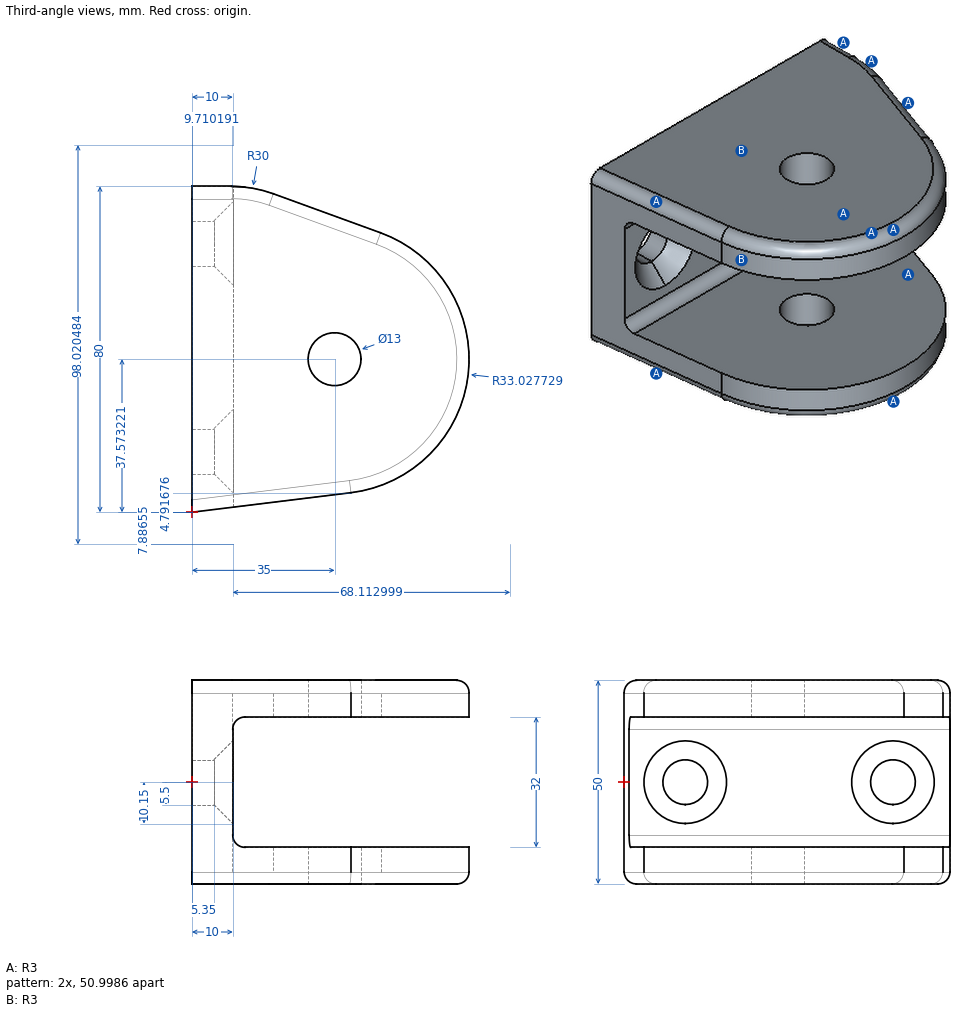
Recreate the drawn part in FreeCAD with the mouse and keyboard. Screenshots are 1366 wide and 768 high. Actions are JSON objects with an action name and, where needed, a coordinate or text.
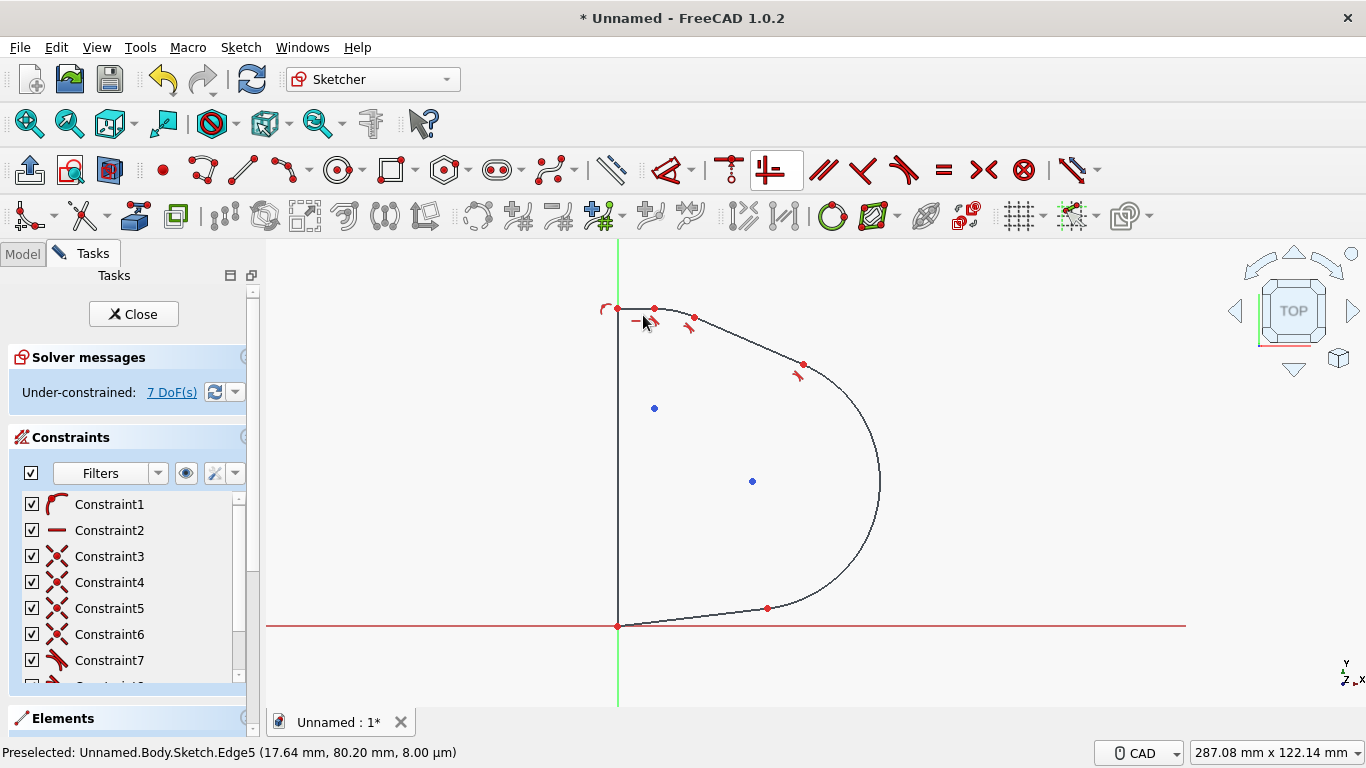
{"action": "left_click", "coordinate": [723, 614]}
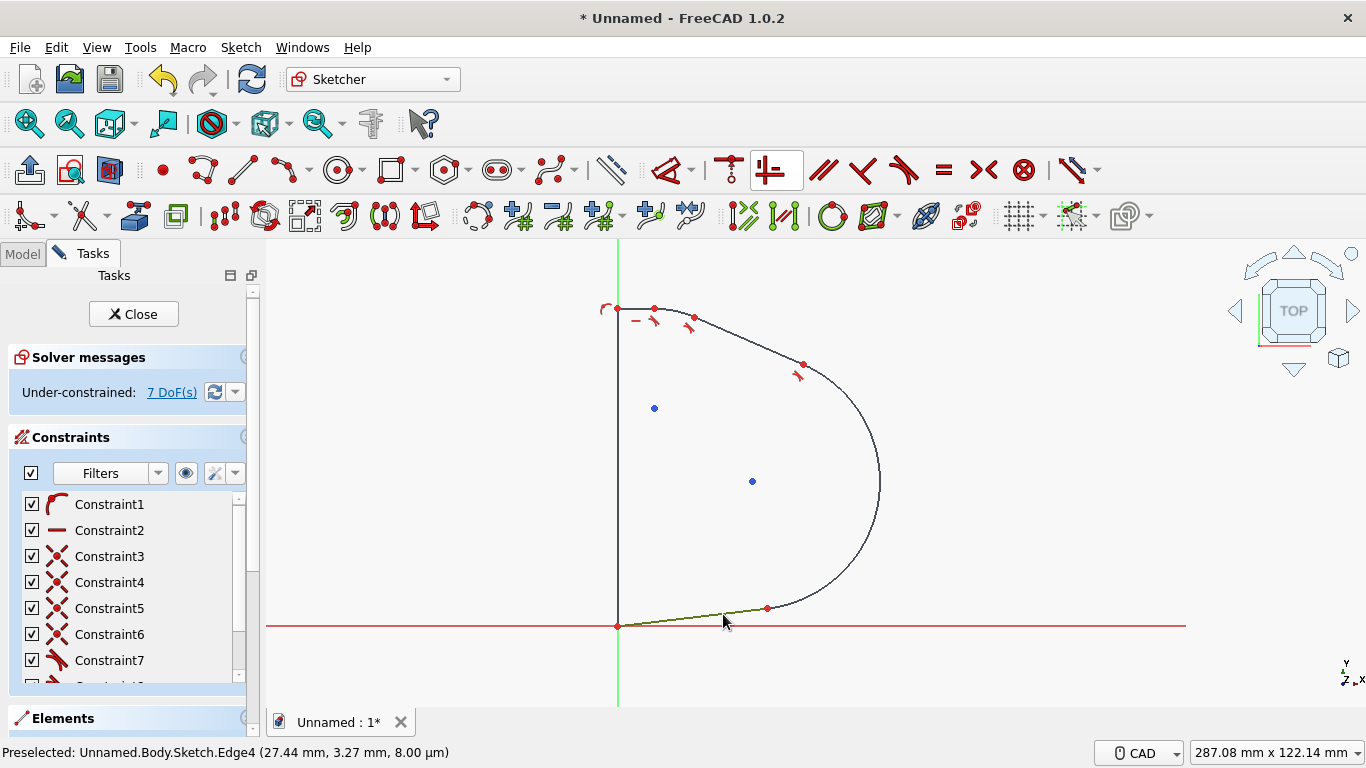
{"action": "left_click", "coordinate": [853, 561]}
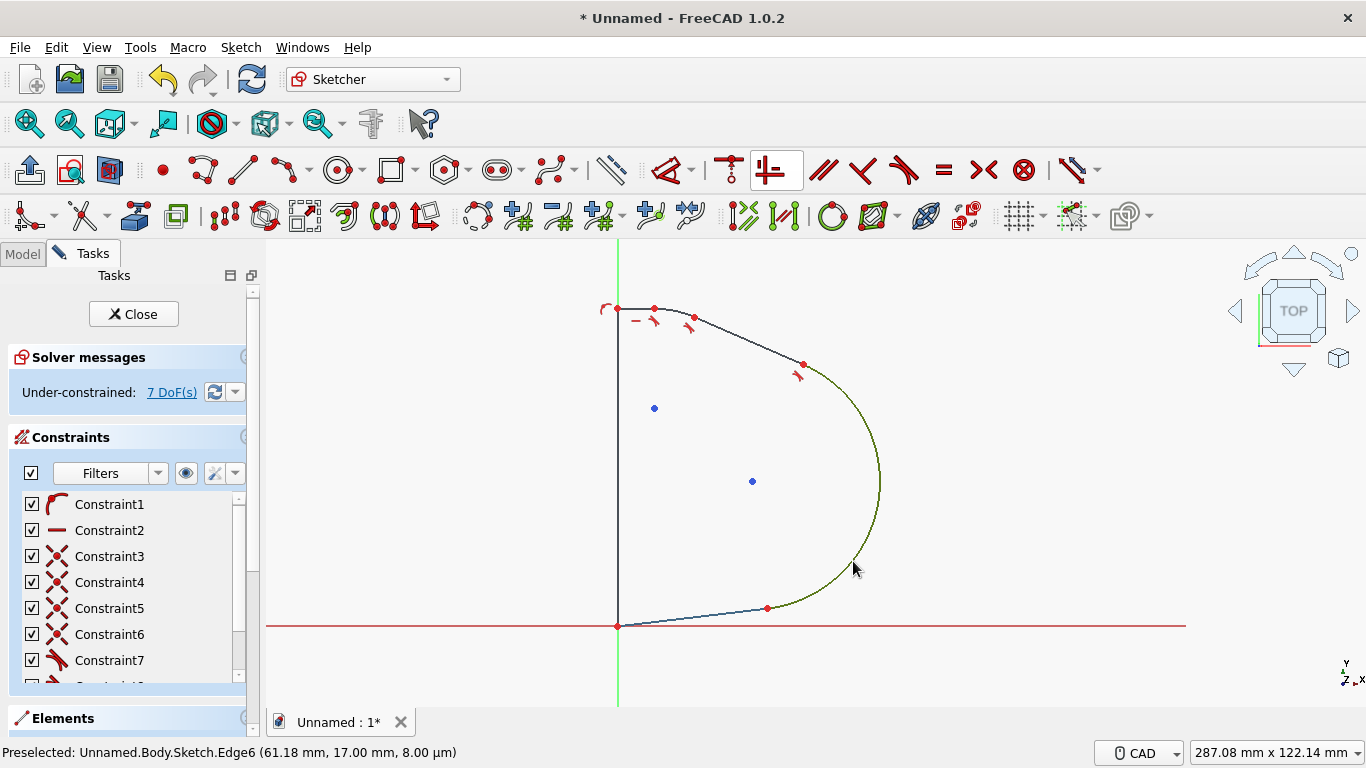
{"action": "left_click", "coordinate": [904, 170]}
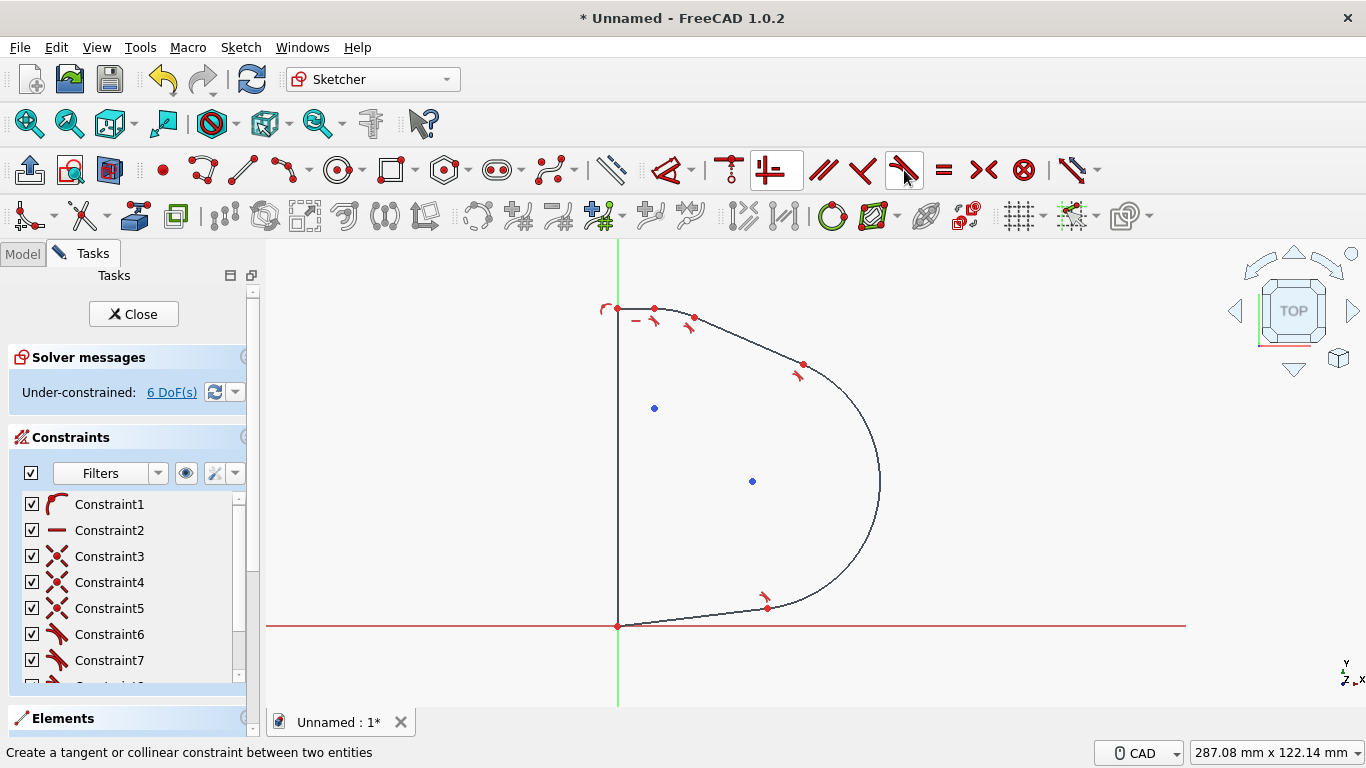
{"action": "left_click", "coordinate": [666, 170]}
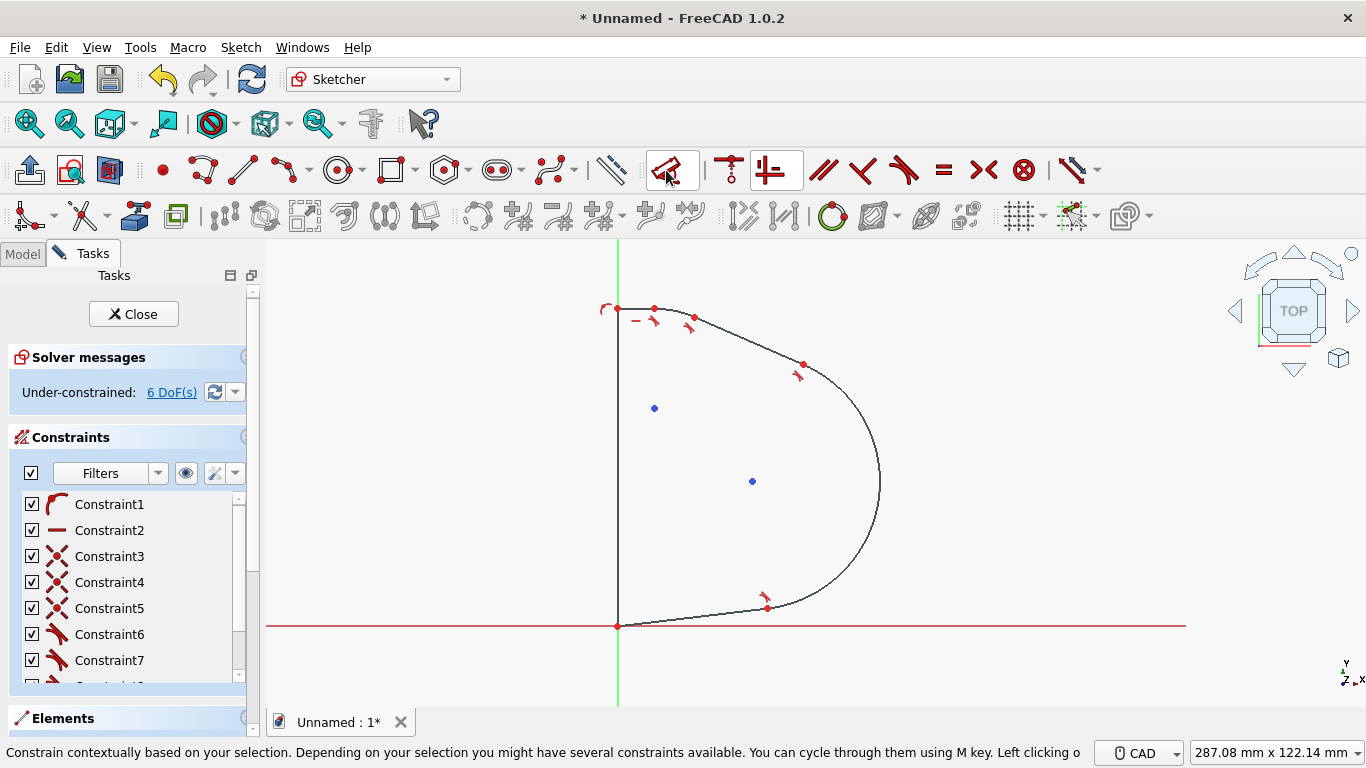
{"action": "left_click", "coordinate": [683, 313]}
{"action": "left_click", "coordinate": [692, 282]}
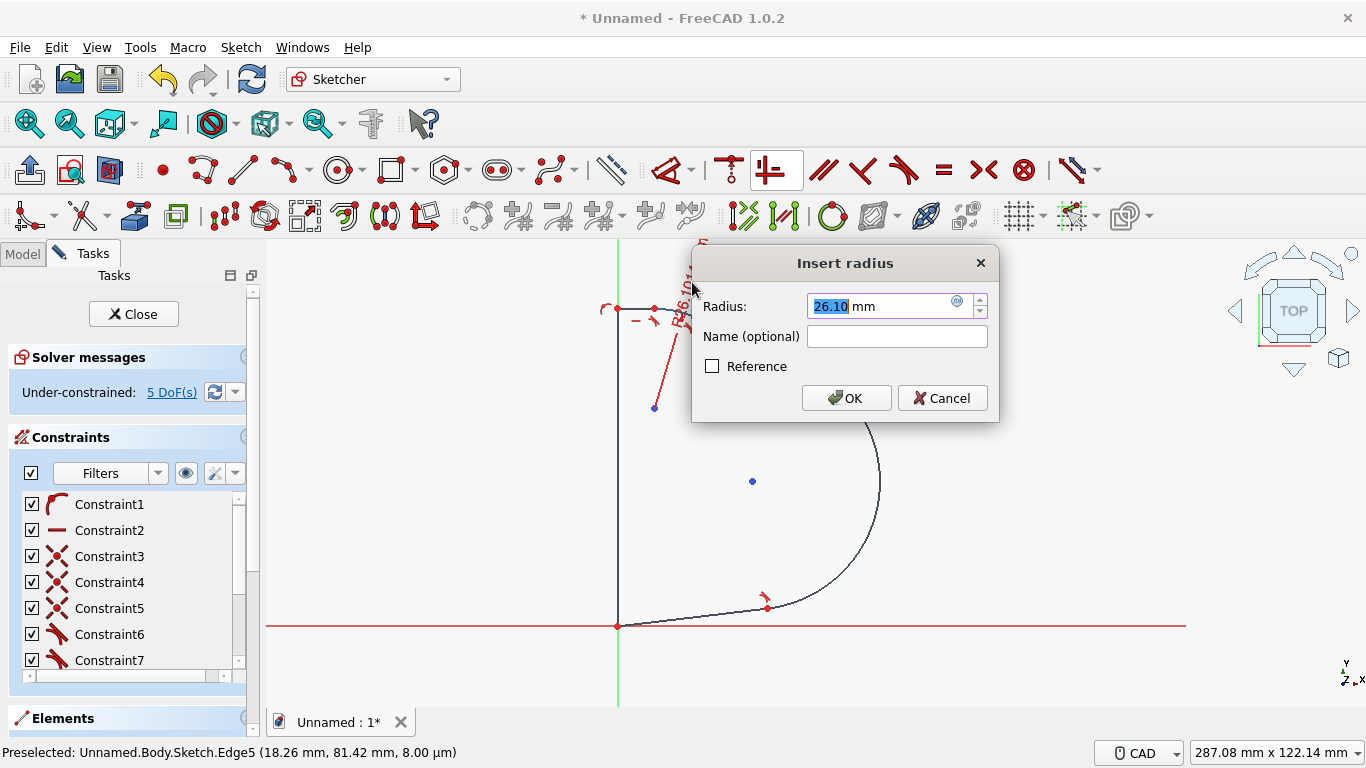
{"action": "type", "text": "30"}
{"action": "key", "text": "Return"}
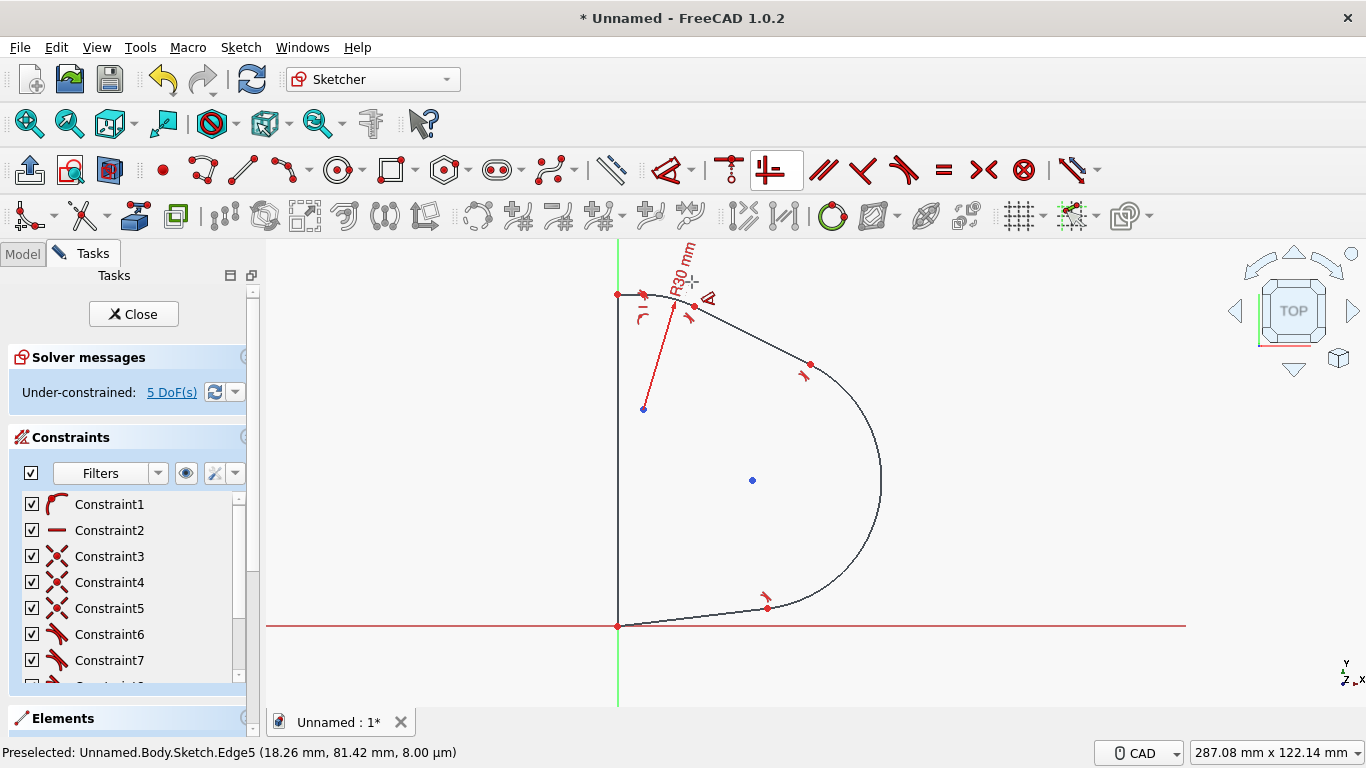
{"action": "left_click", "coordinate": [852, 562]}
{"action": "left_click", "coordinate": [877, 582]}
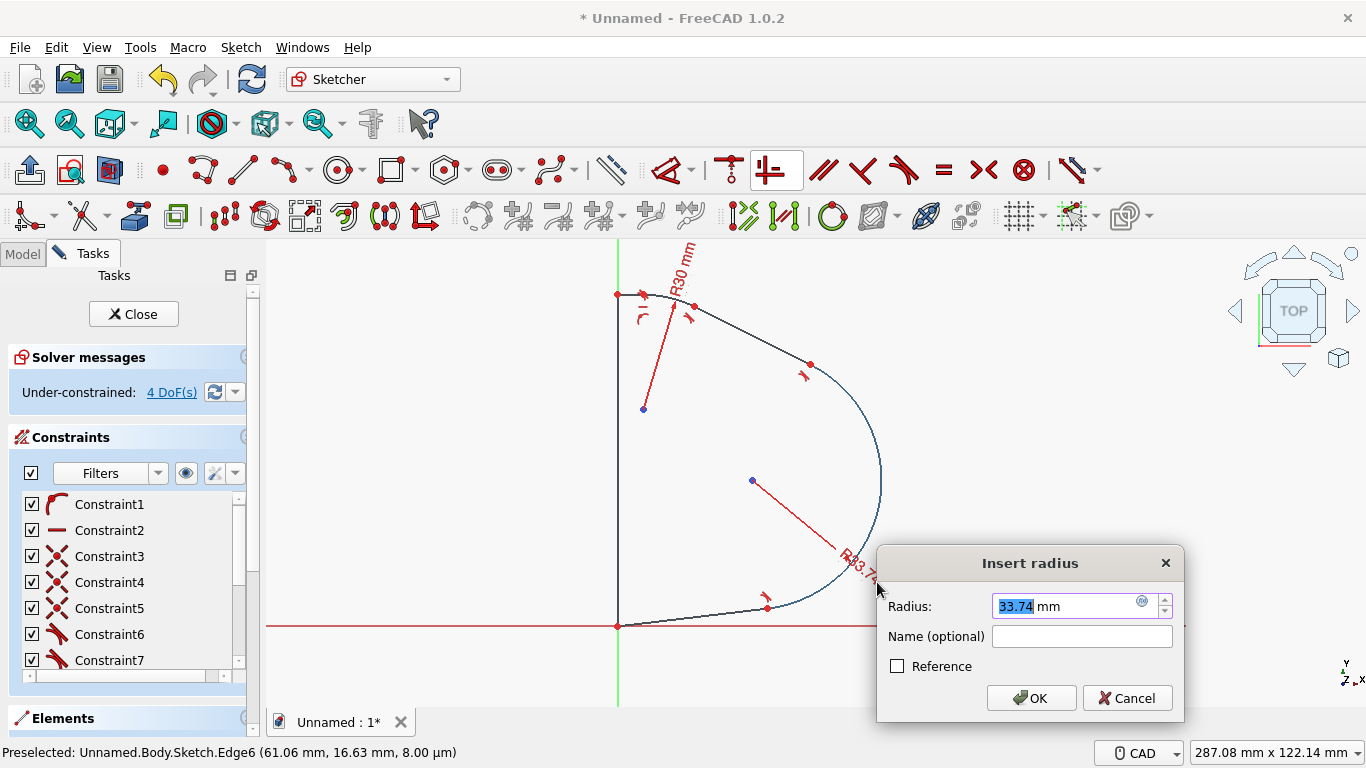
{"action": "type", "text": "33.027729"}
{"action": "key", "text": "Return"}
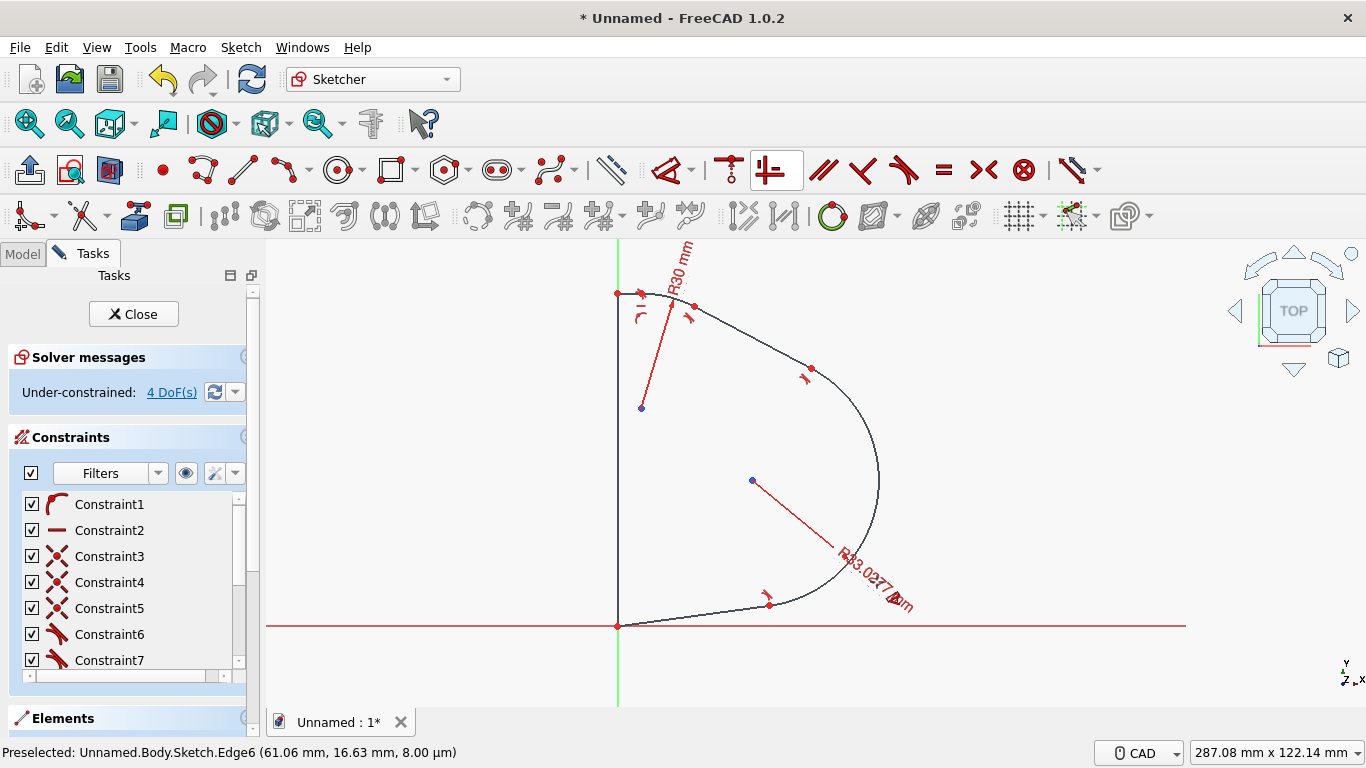
{"action": "left_click", "coordinate": [618, 393]}
{"action": "left_click", "coordinate": [584, 460]}